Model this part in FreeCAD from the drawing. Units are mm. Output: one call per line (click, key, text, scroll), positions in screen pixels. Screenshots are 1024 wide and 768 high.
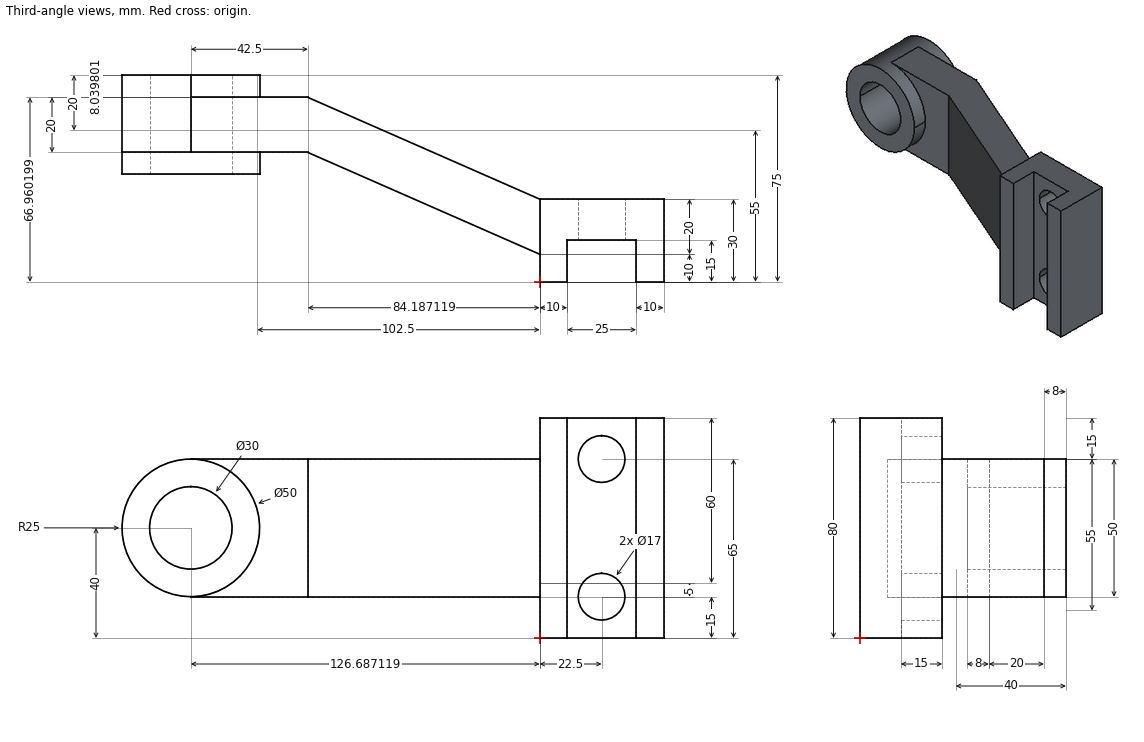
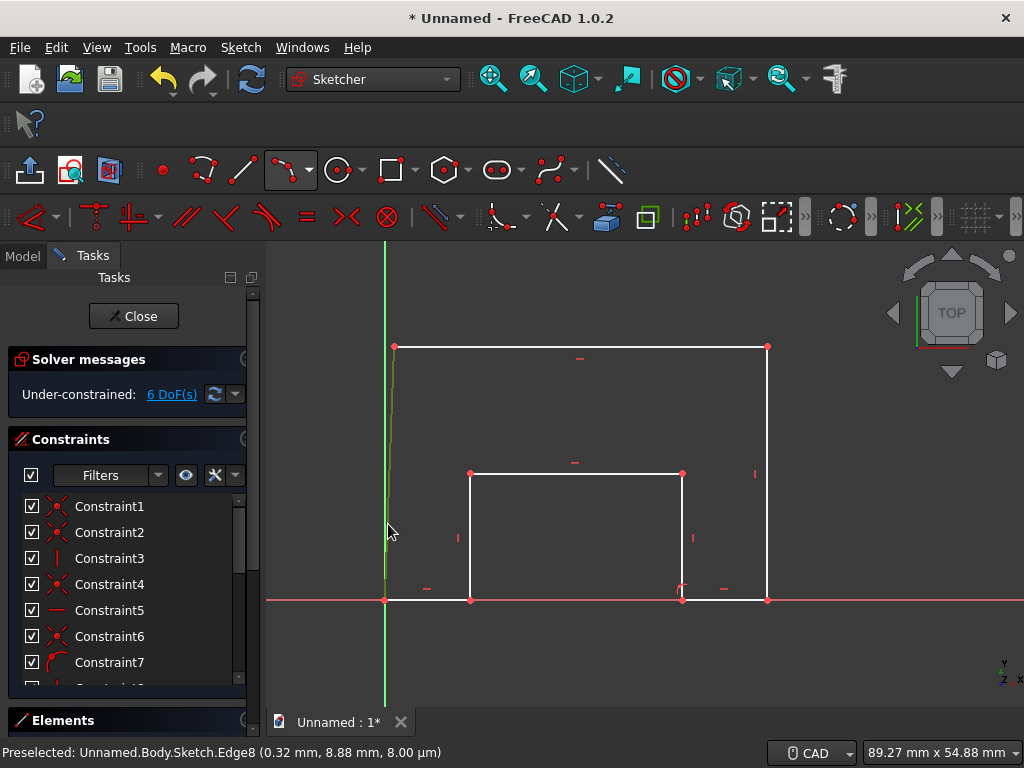
key(v)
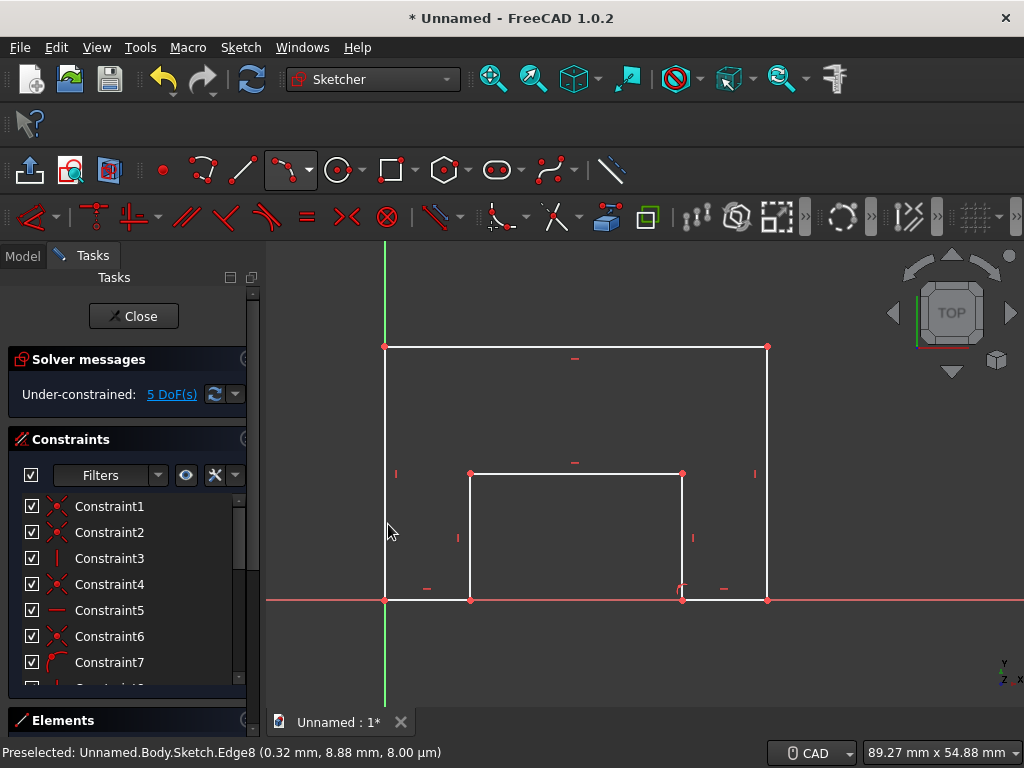
click(410, 600)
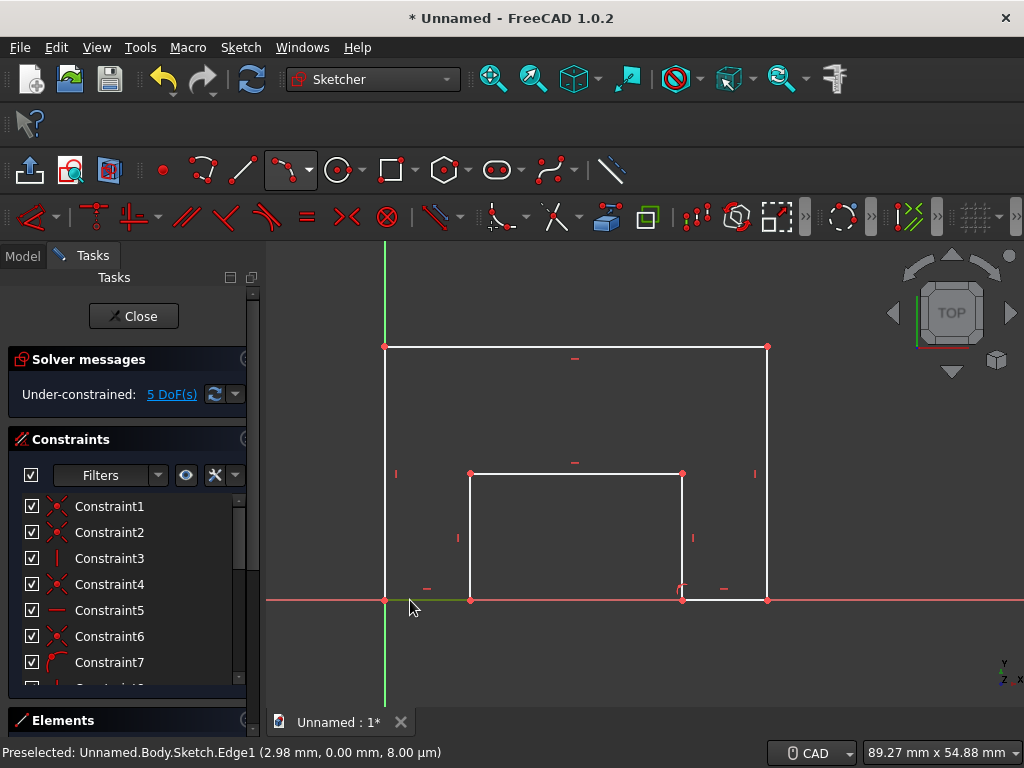
key(l)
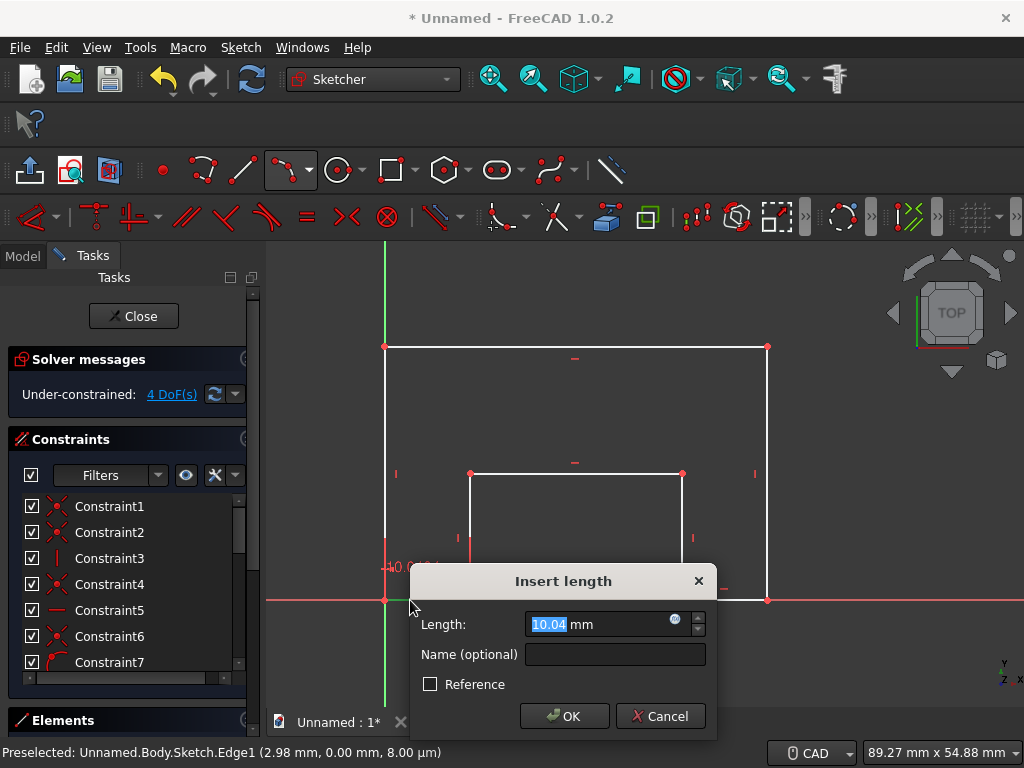
text(10)
key(Return)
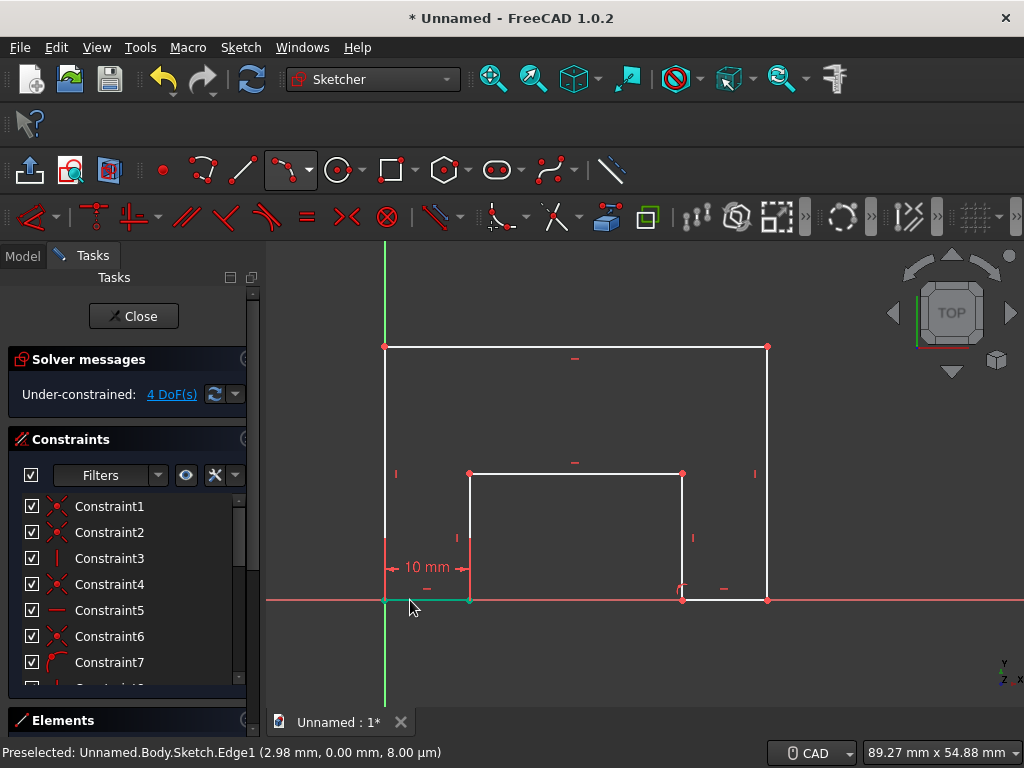
click(470, 562)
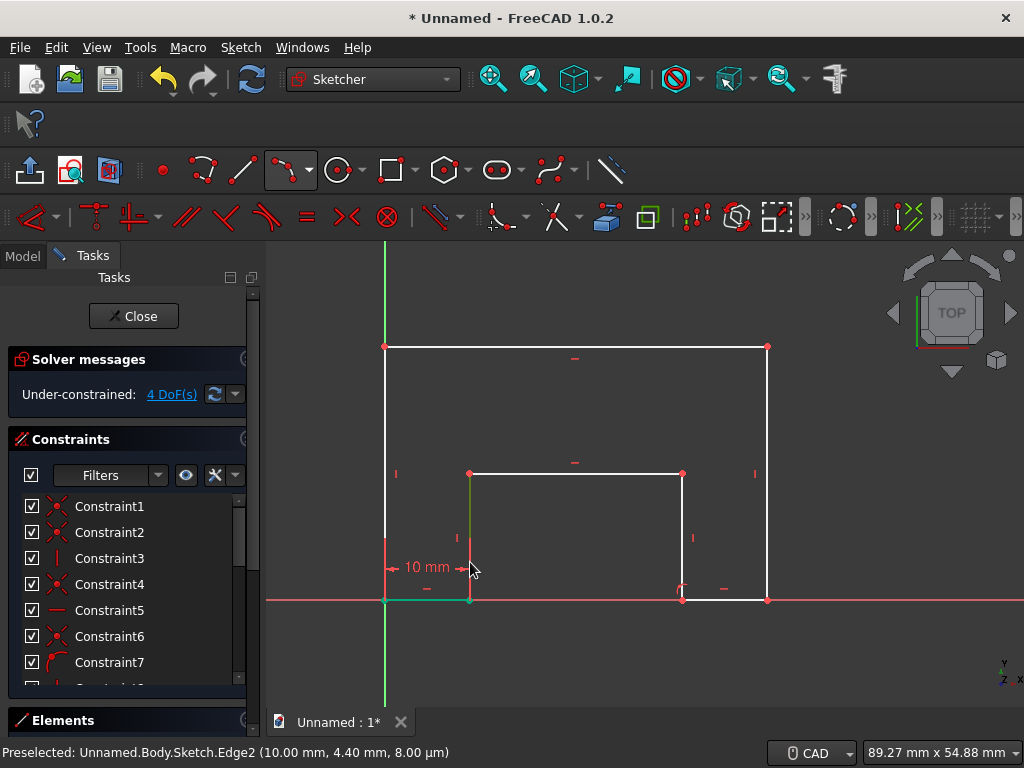
key(i)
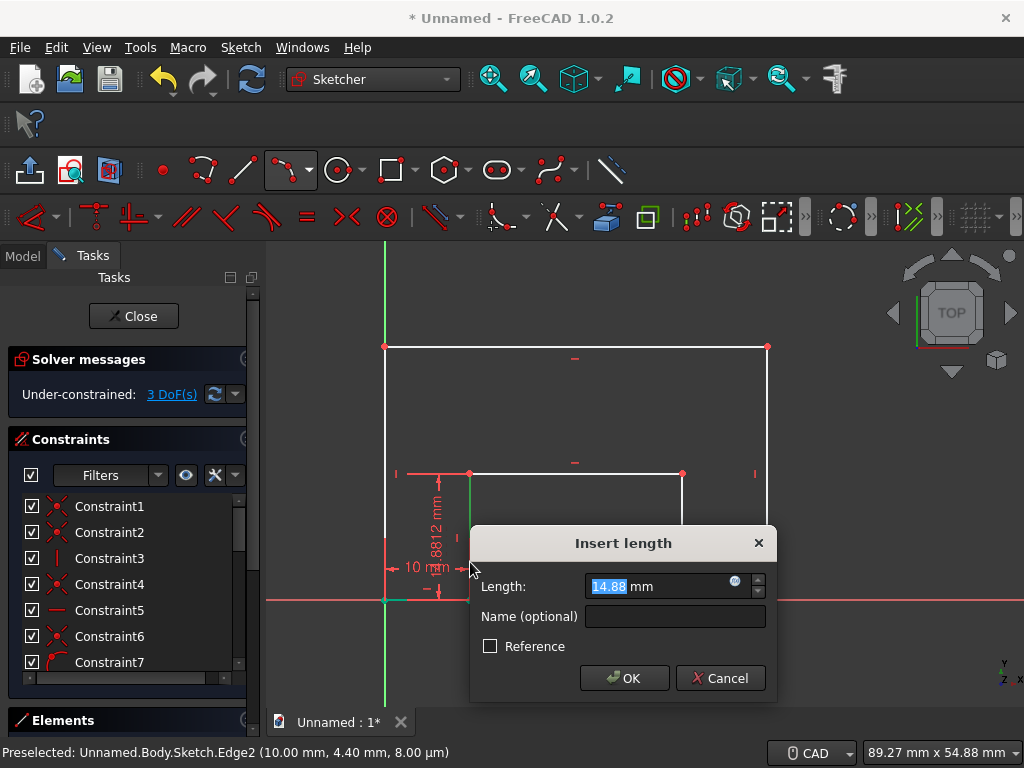
text(15)
key(Return)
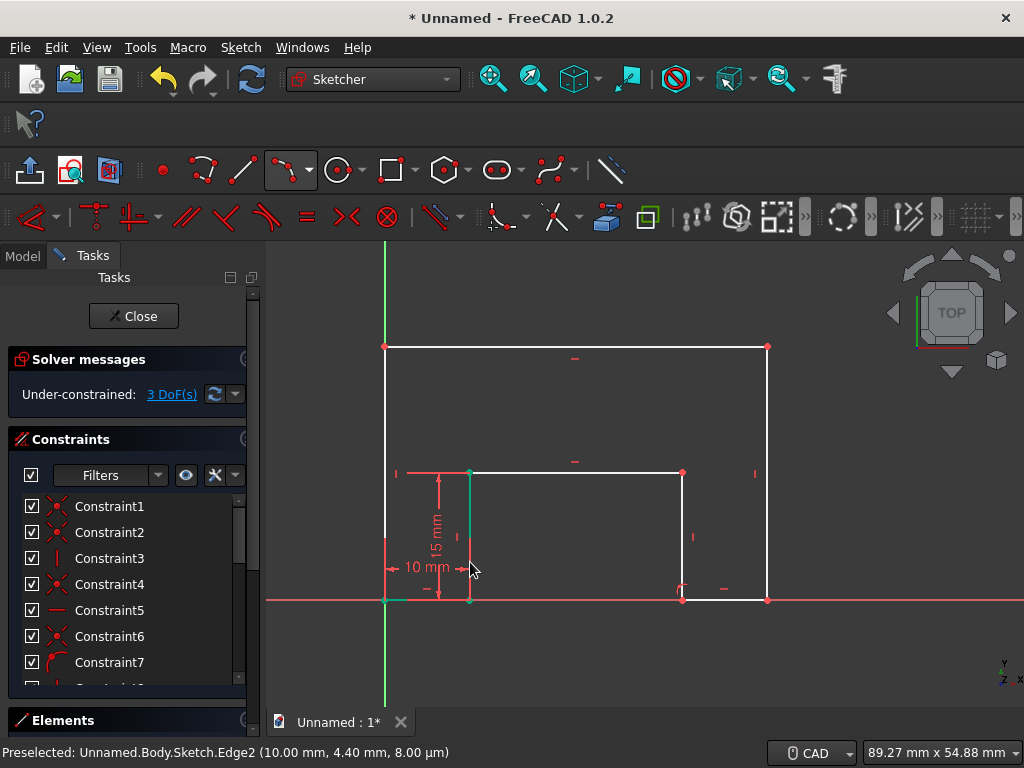
click(533, 473)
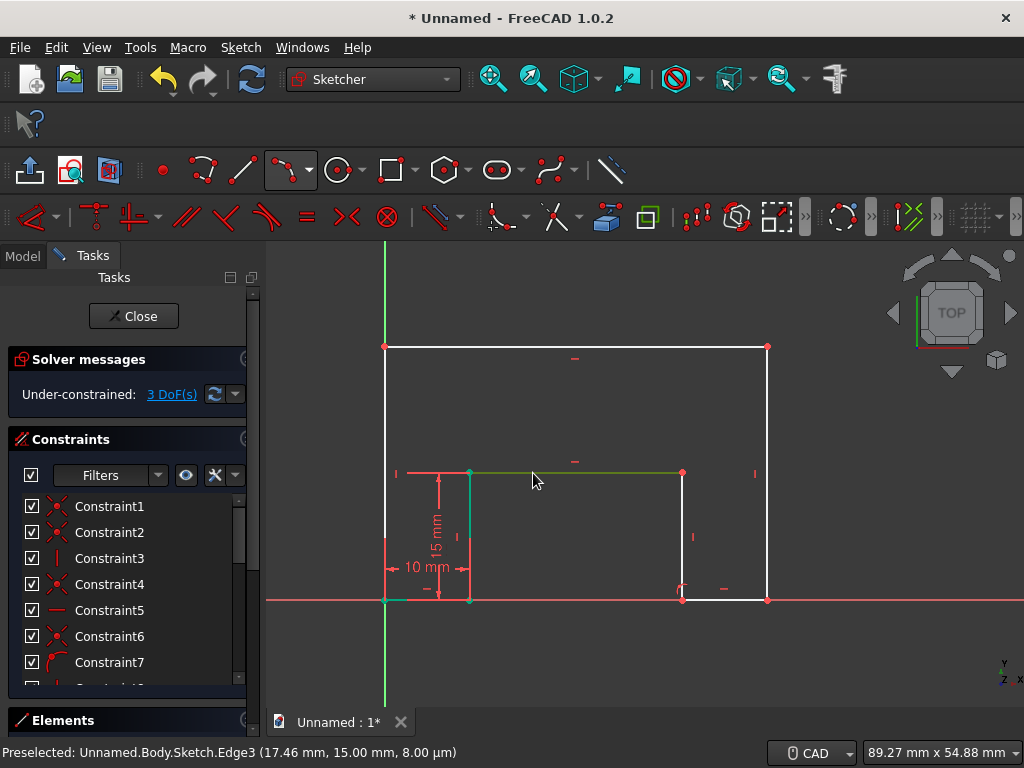
key(l)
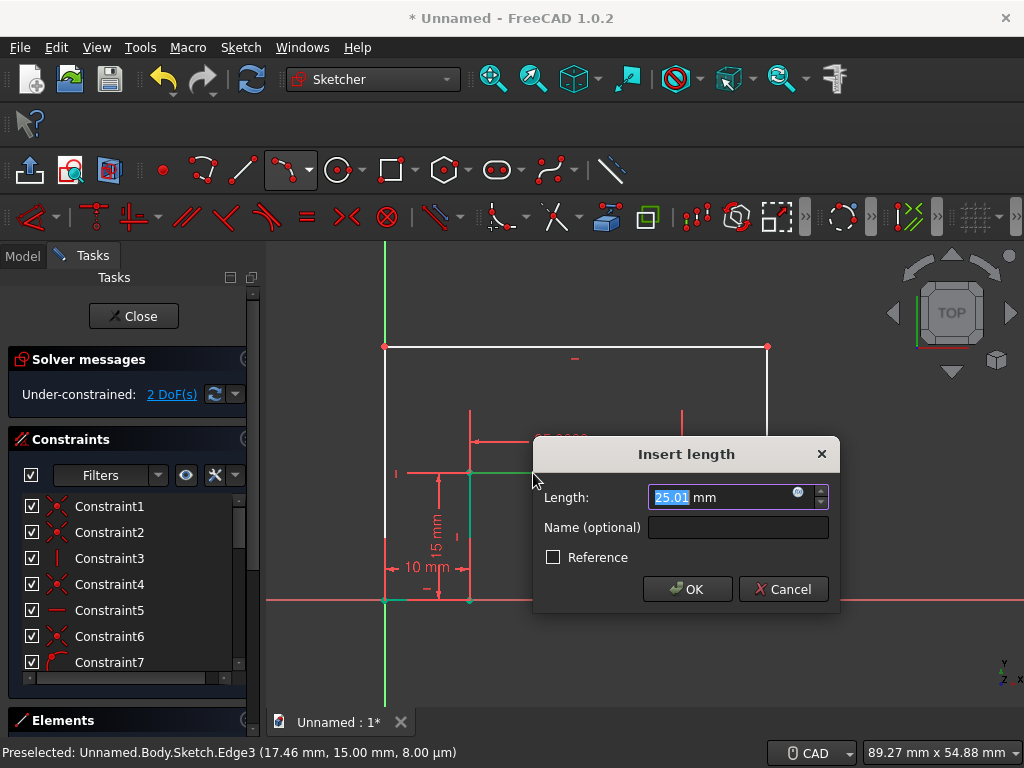
text(25)
key(Return)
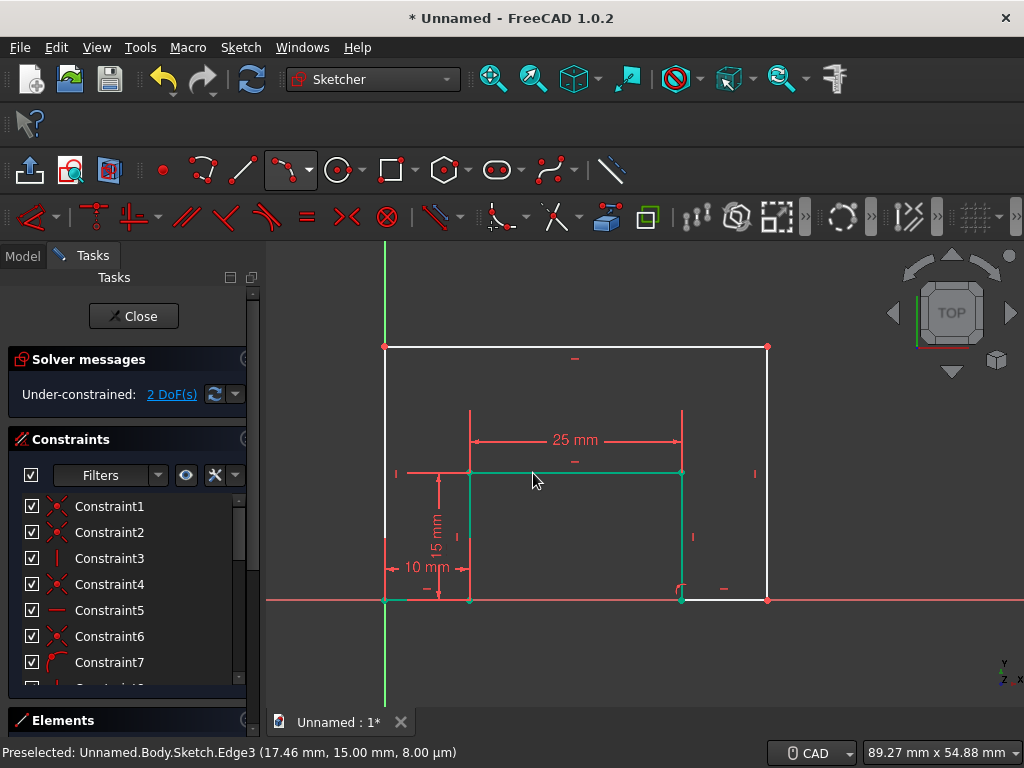
click(707, 600)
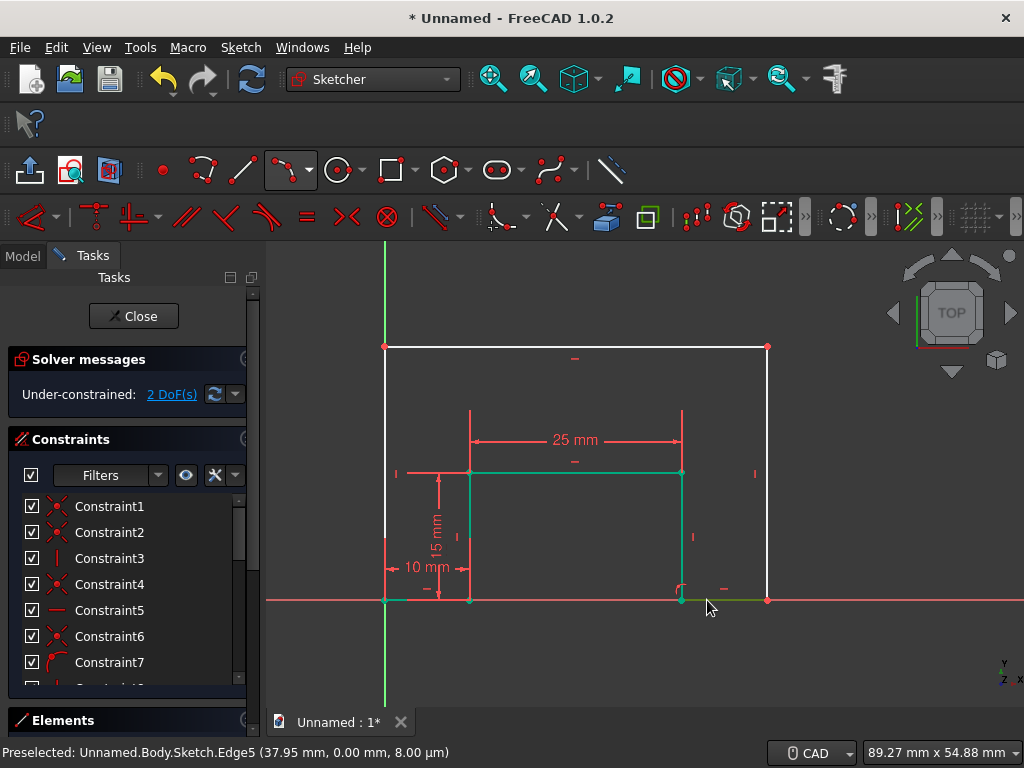
key(l)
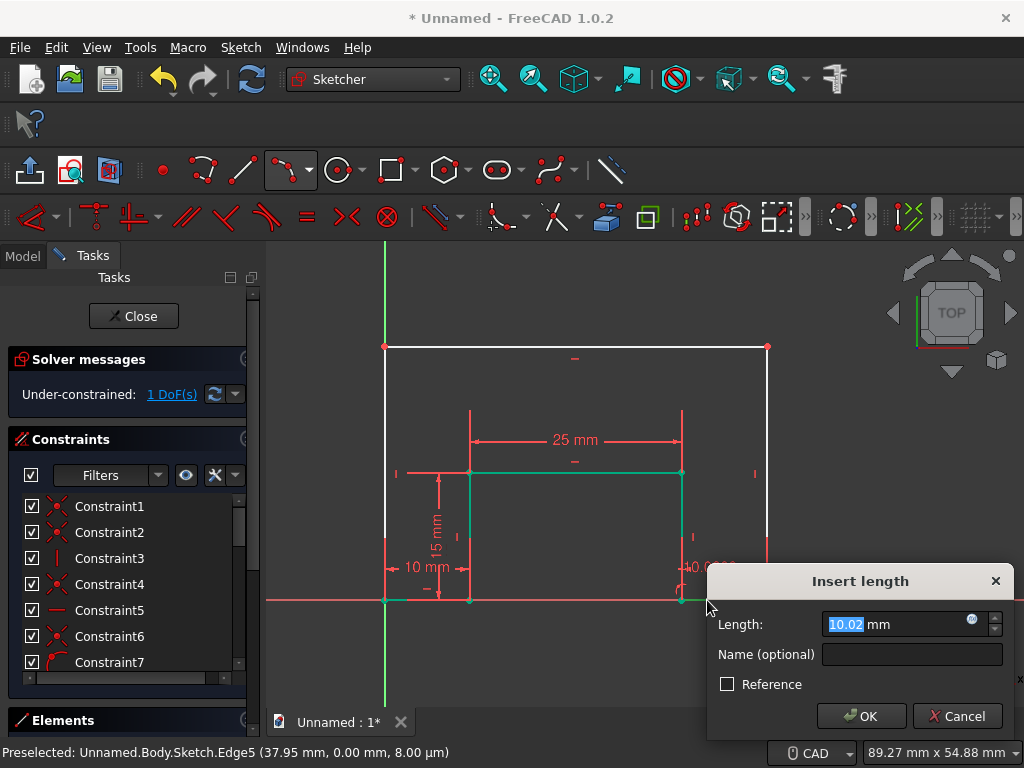
text(10)
key(Return)